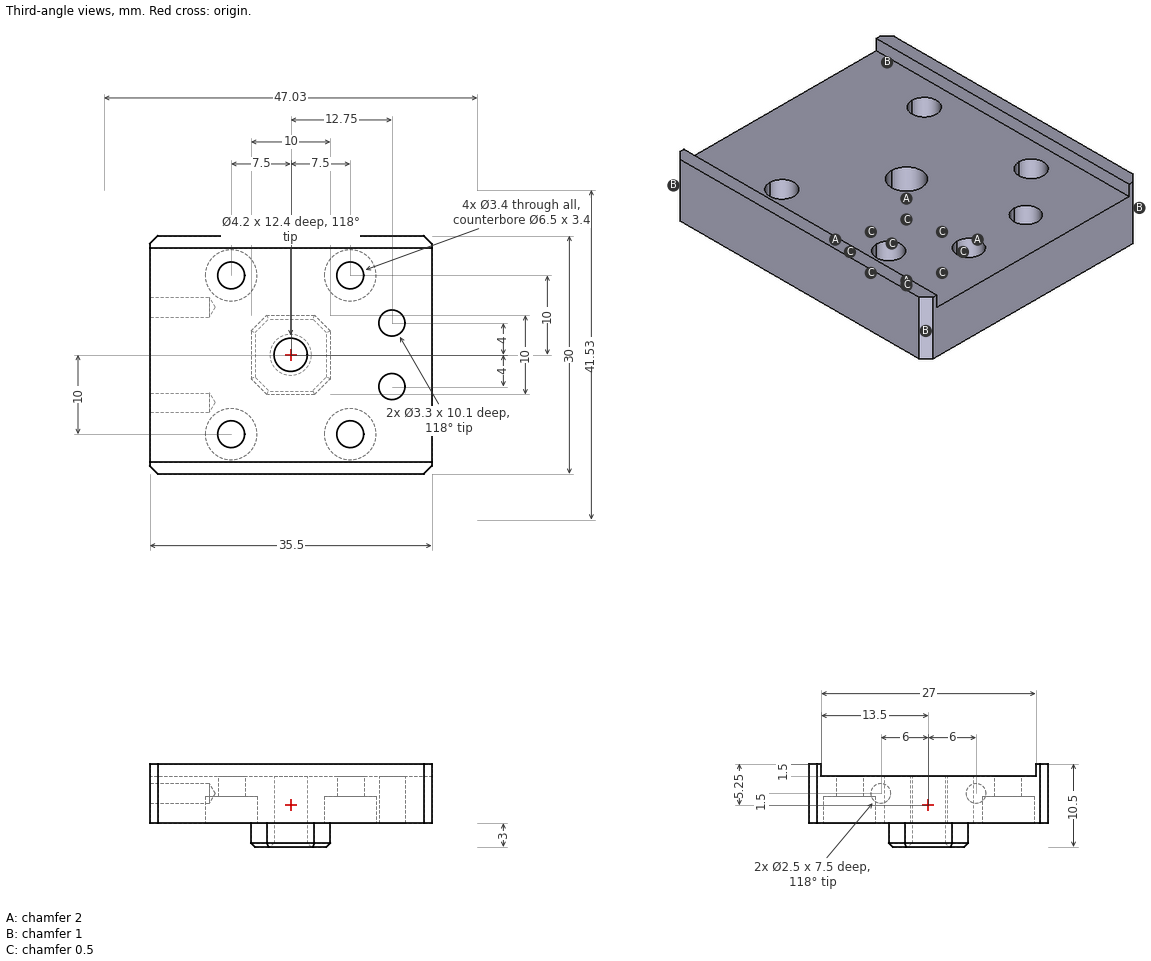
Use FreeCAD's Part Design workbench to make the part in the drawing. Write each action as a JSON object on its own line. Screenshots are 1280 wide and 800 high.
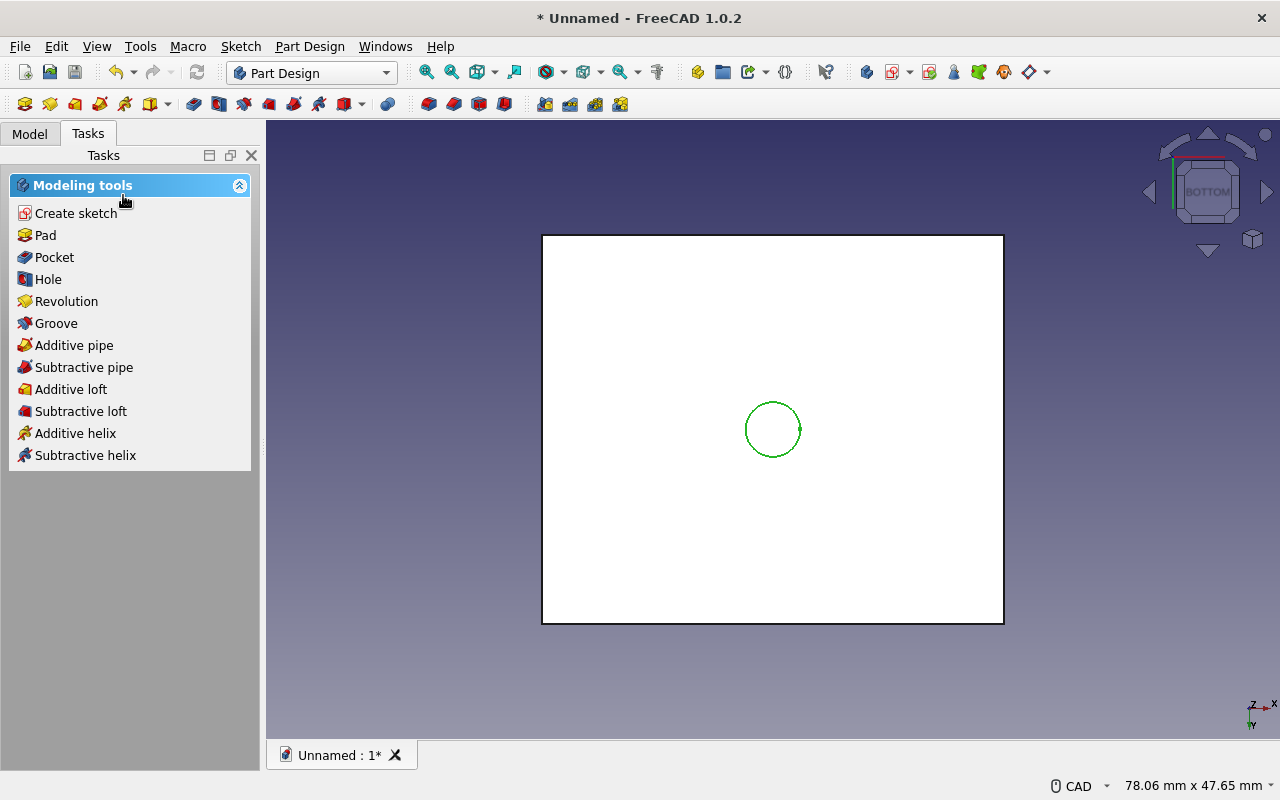
{"action": "left_click", "coordinate": [219, 104]}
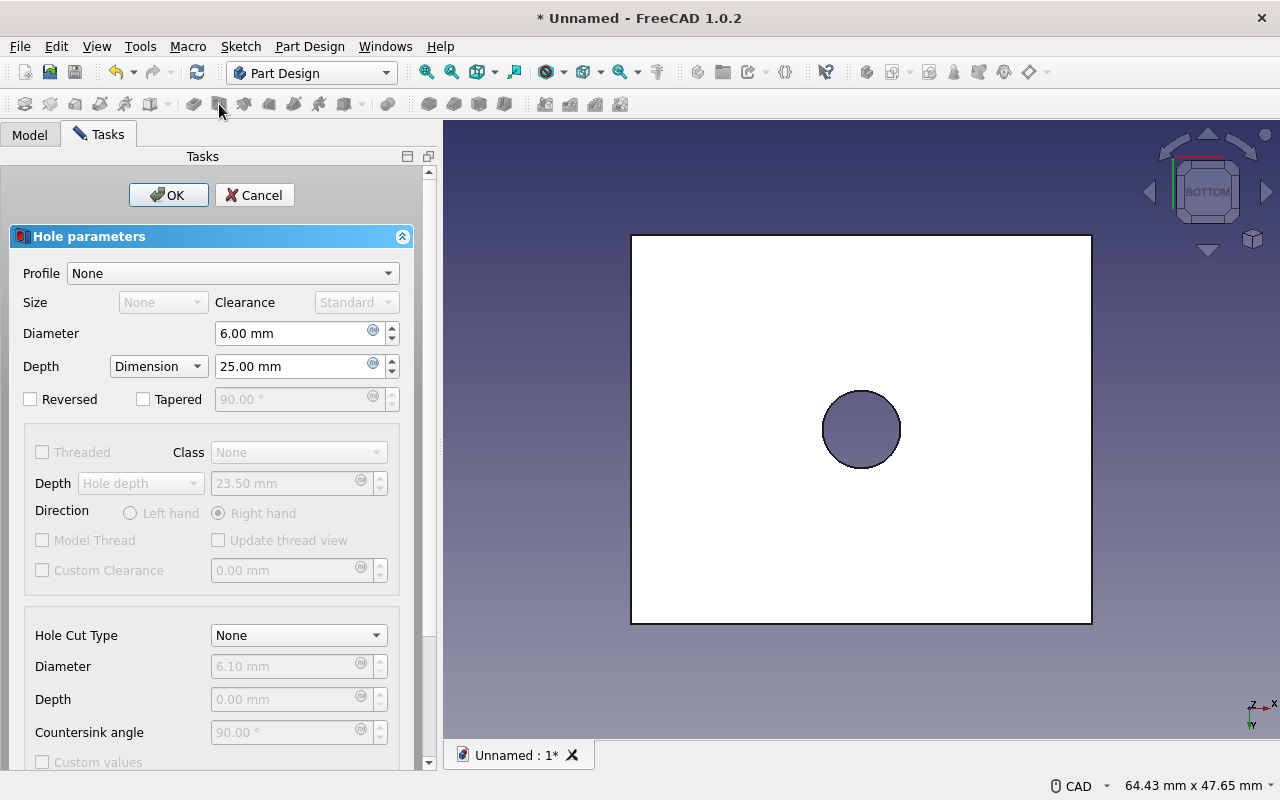
{"action": "triple_click", "coordinate": [300, 334]}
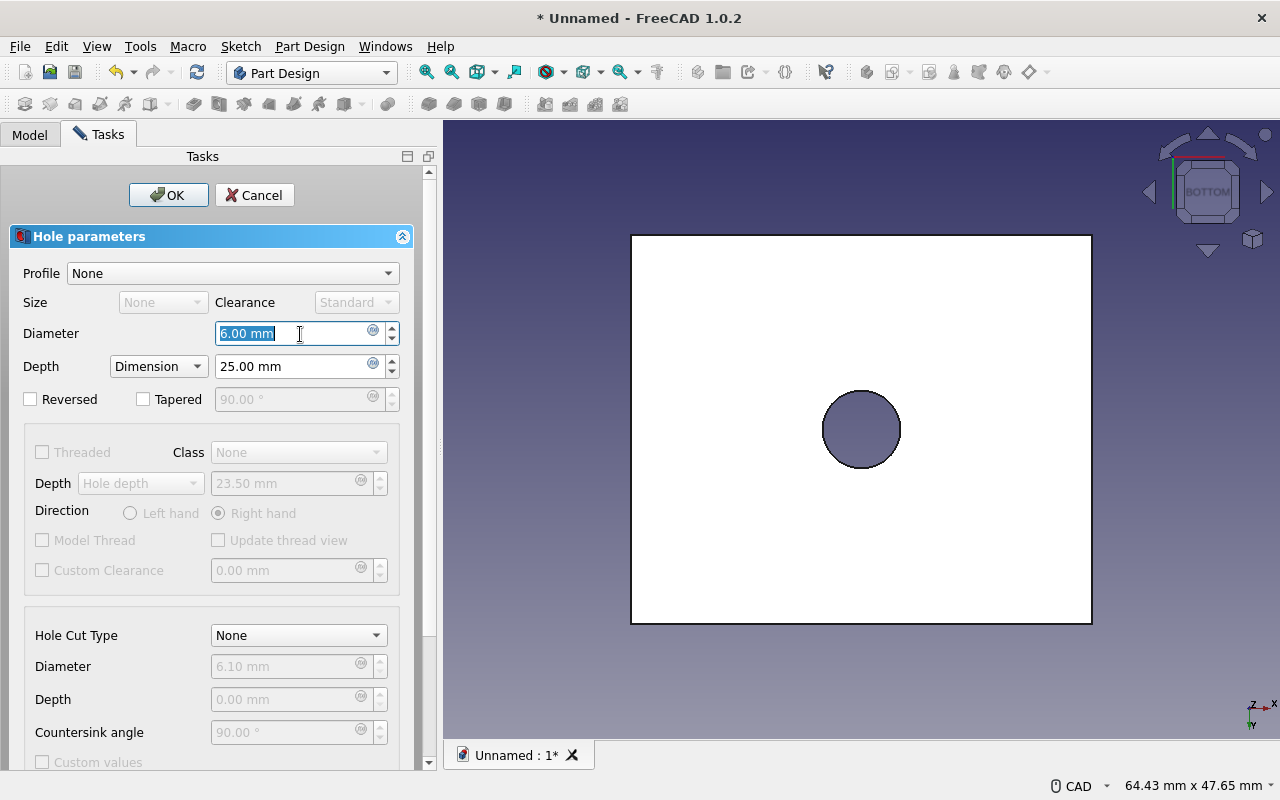
{"action": "type", "text": "4.2"}
{"action": "key", "text": "Tab"}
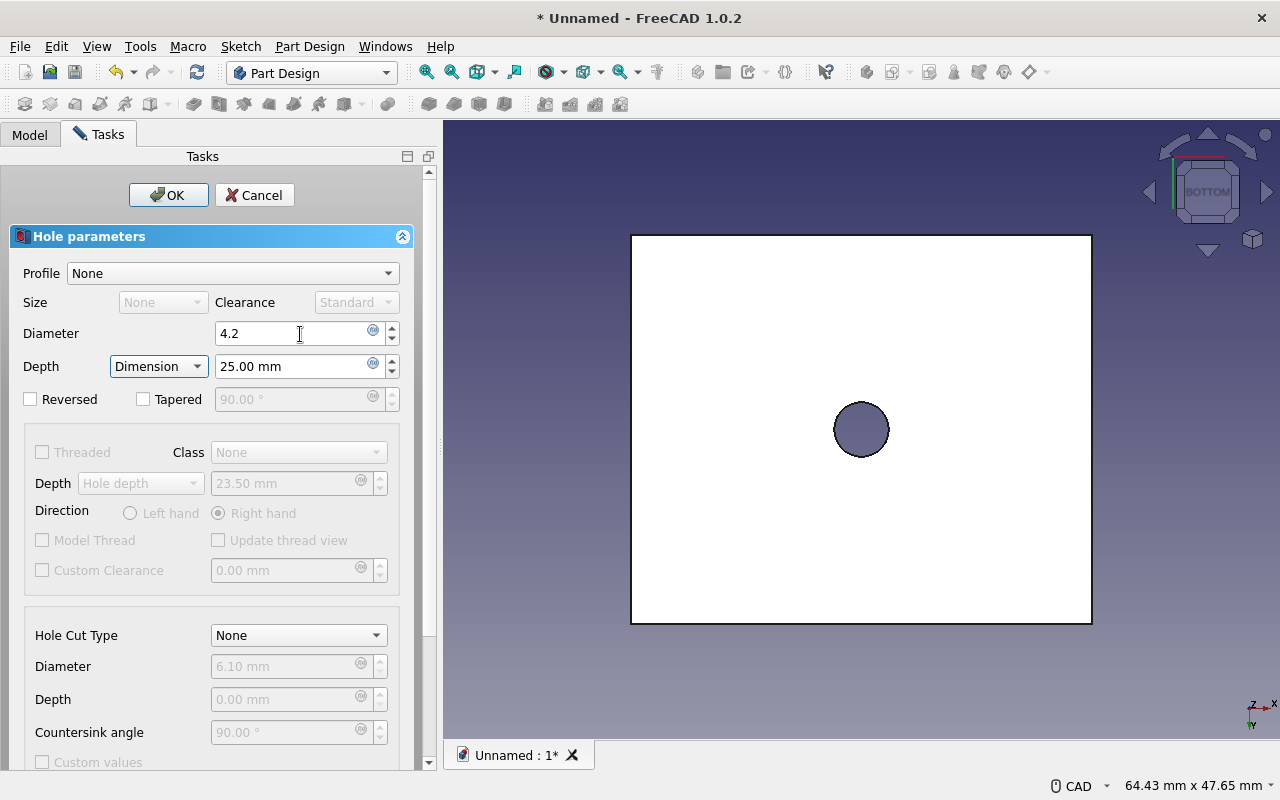
{"action": "triple_click", "coordinate": [300, 366]}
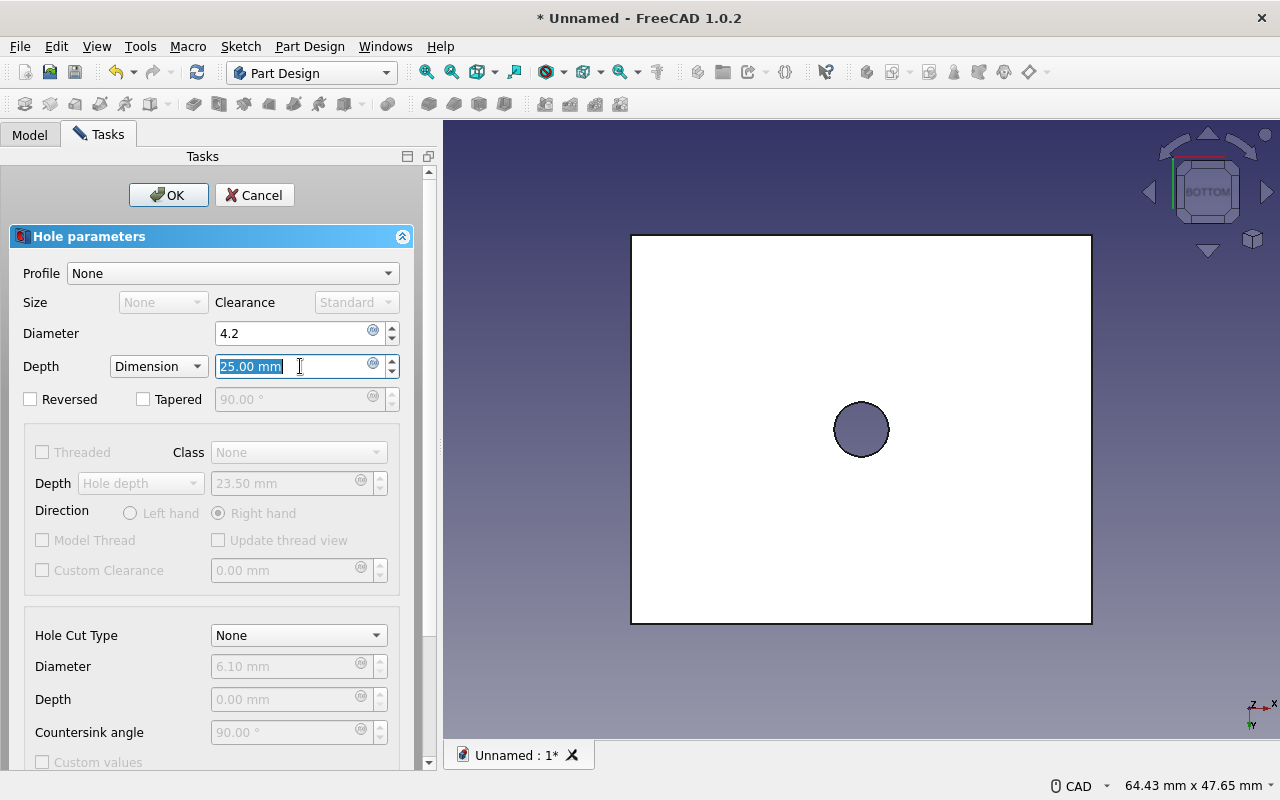
{"action": "type", "text": "12.4"}
{"action": "key", "text": "Tab"}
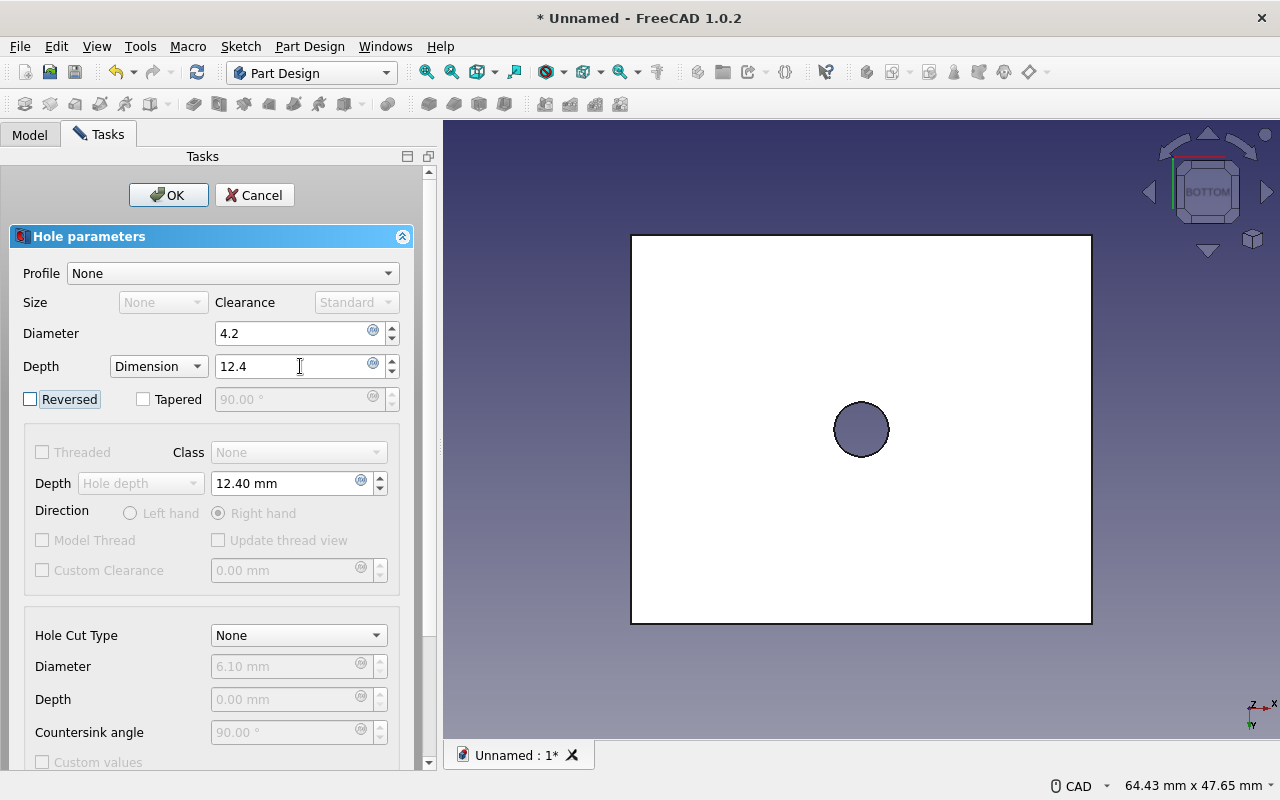
{"action": "left_click", "coordinate": [169, 195]}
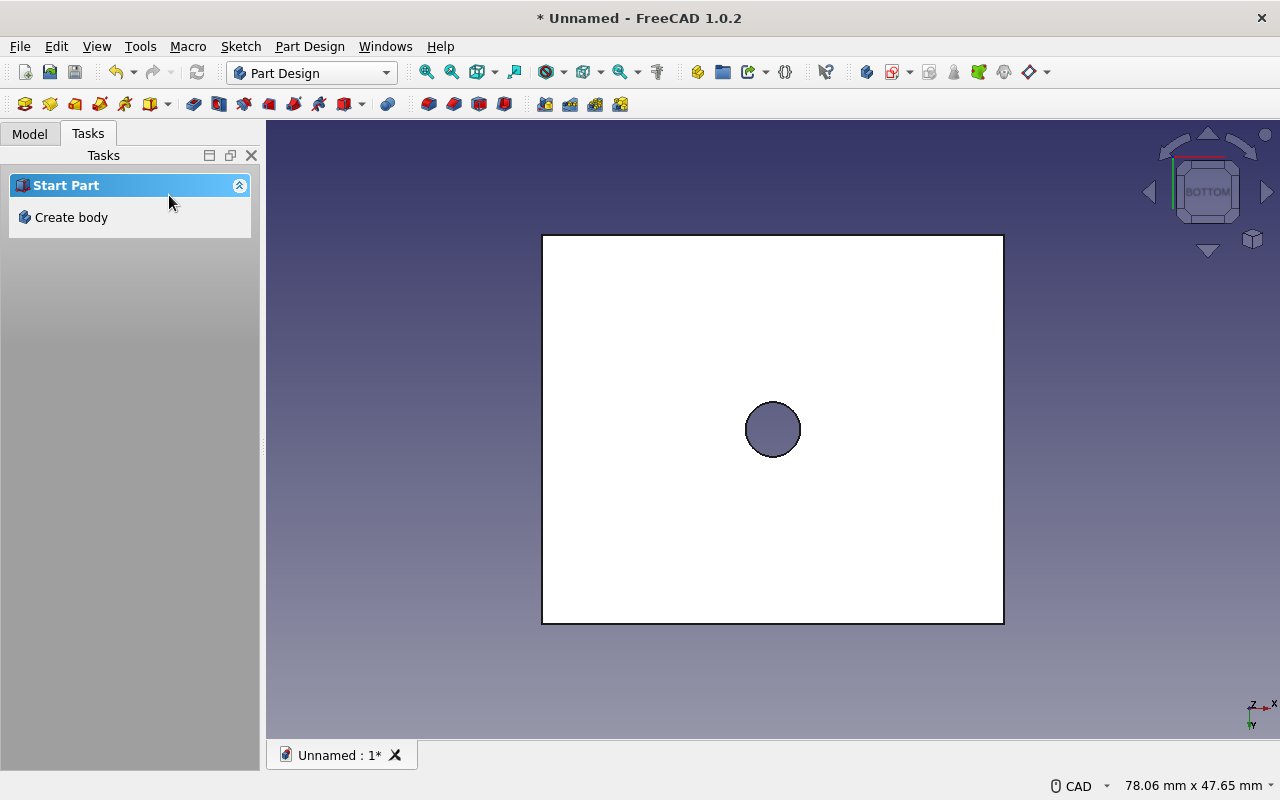
{"action": "left_click", "coordinate": [905, 484]}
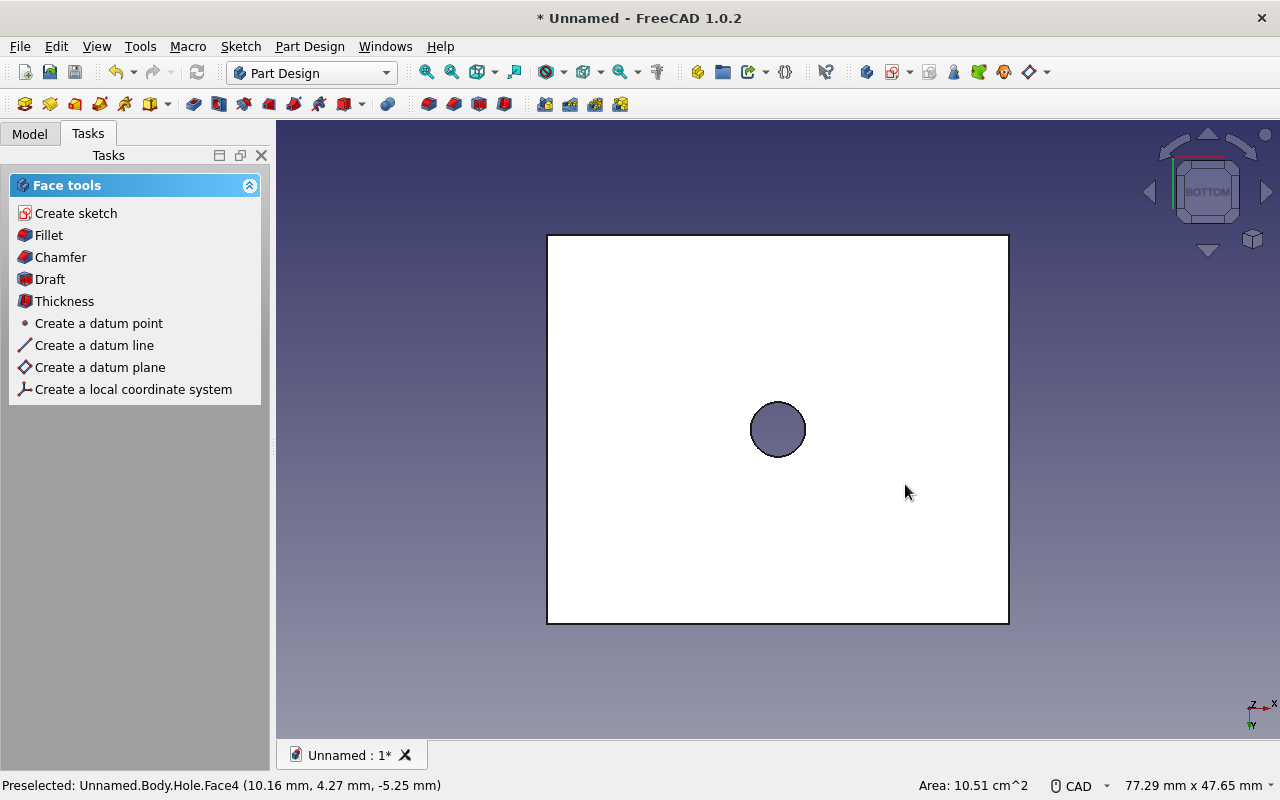
{"action": "left_click", "coordinate": [892, 72]}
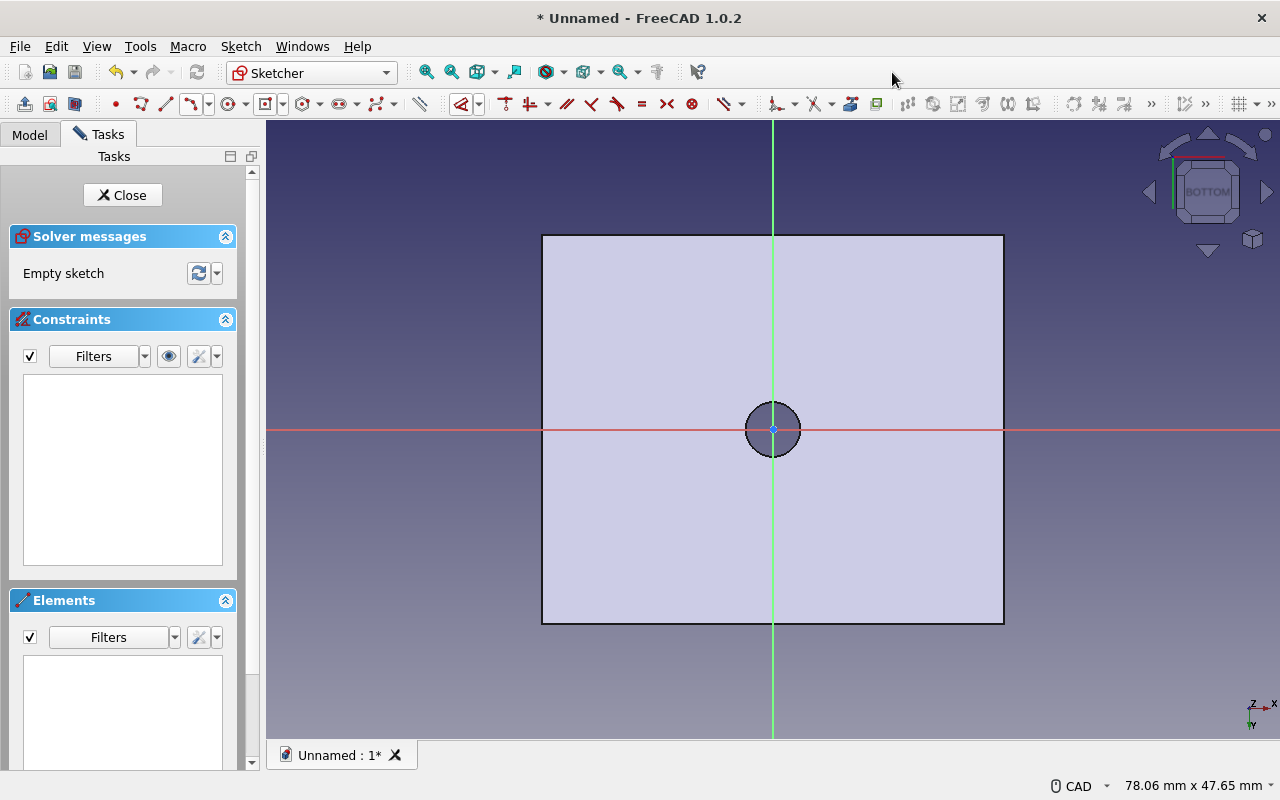
{"action": "scroll", "coordinate": [565, 429], "scroll_direction": "down", "scroll_amount": 2}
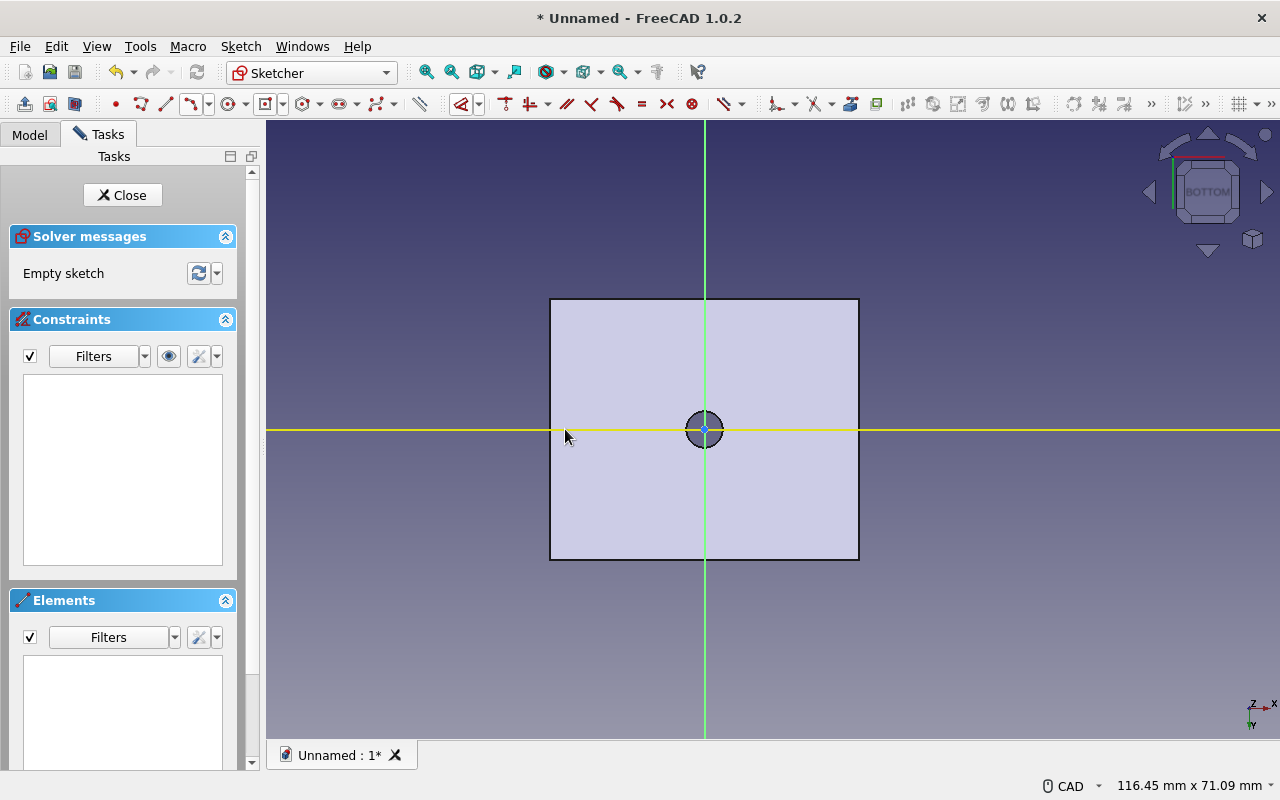
{"action": "left_click", "coordinate": [264, 104]}